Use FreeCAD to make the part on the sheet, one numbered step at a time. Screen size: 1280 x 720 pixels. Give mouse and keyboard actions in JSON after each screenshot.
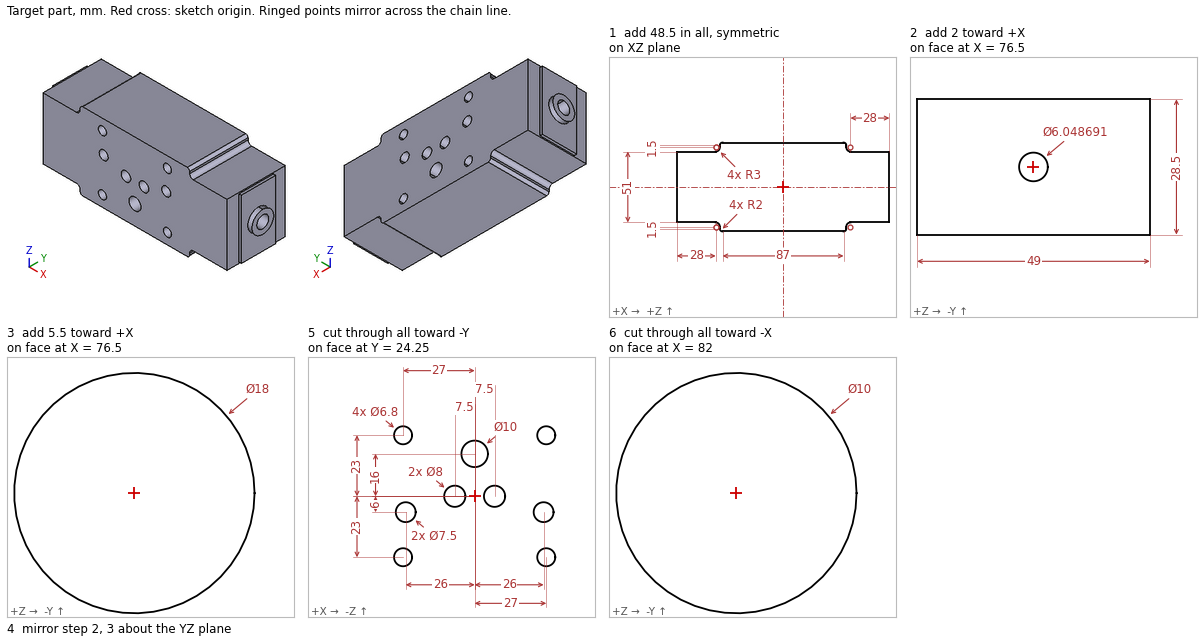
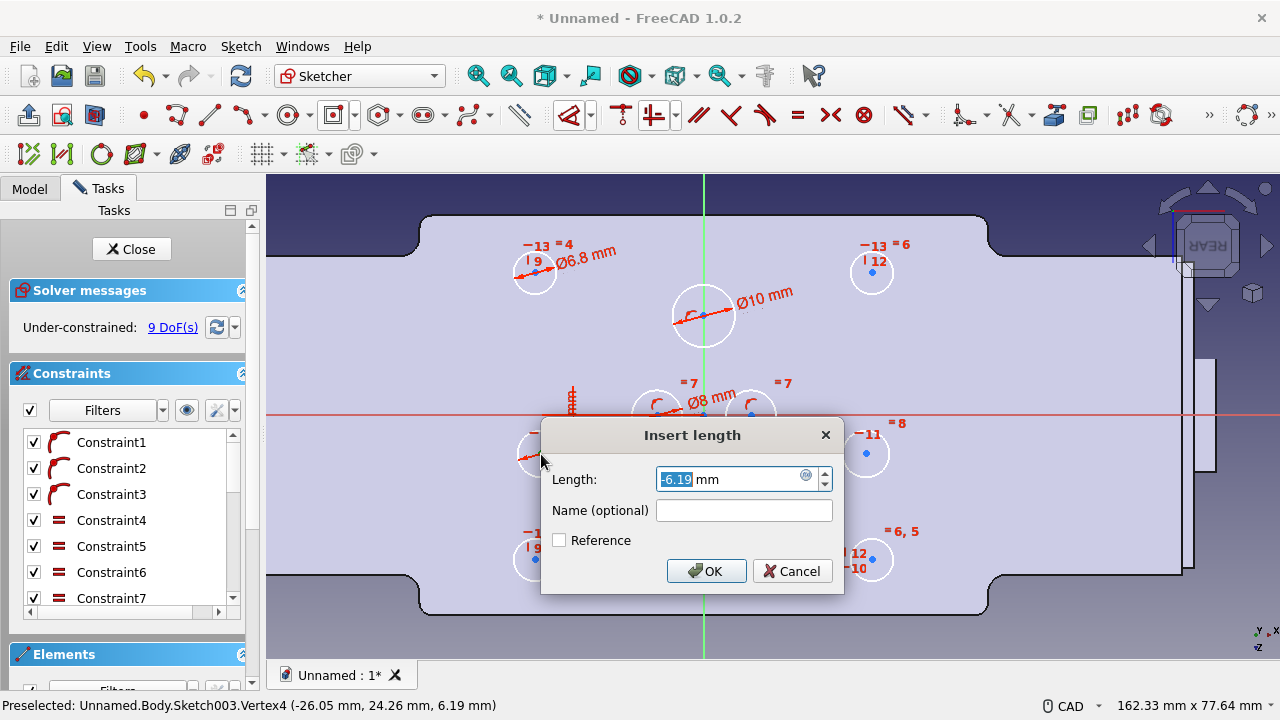
{"action": "type", "text": "-6"}
{"action": "key", "text": "Return"}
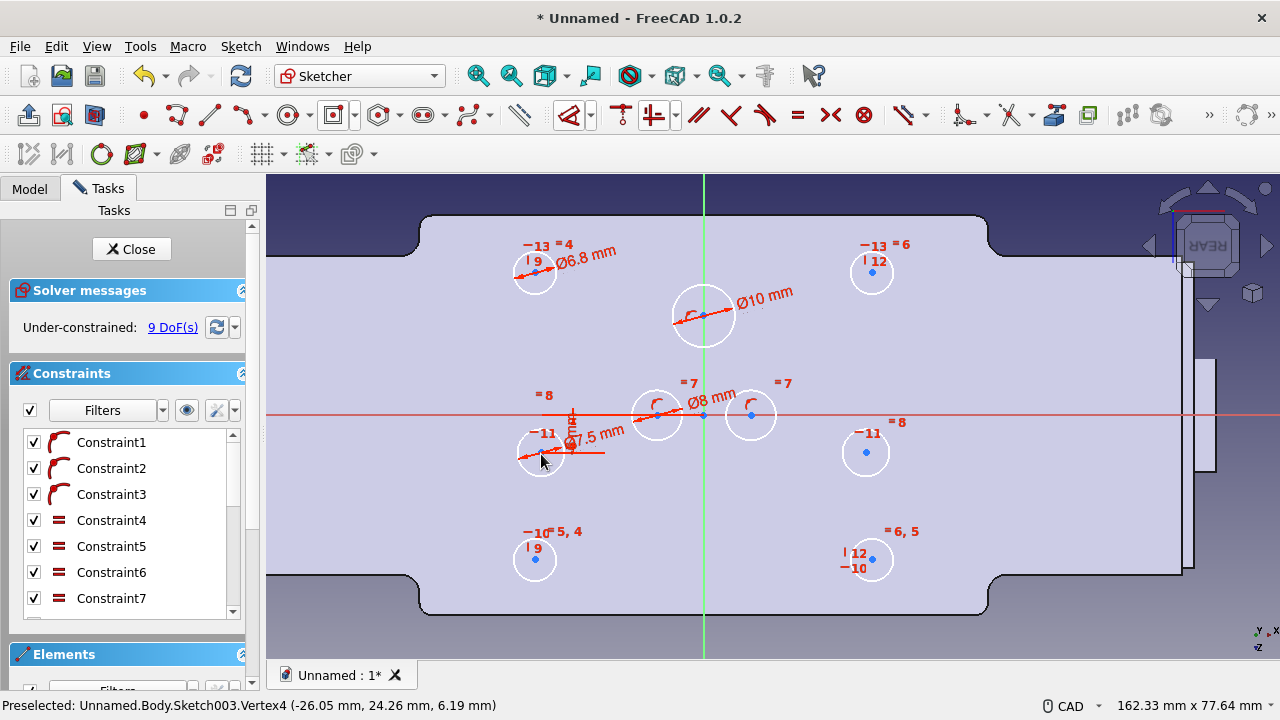
{"action": "left_click", "coordinate": [535, 273]}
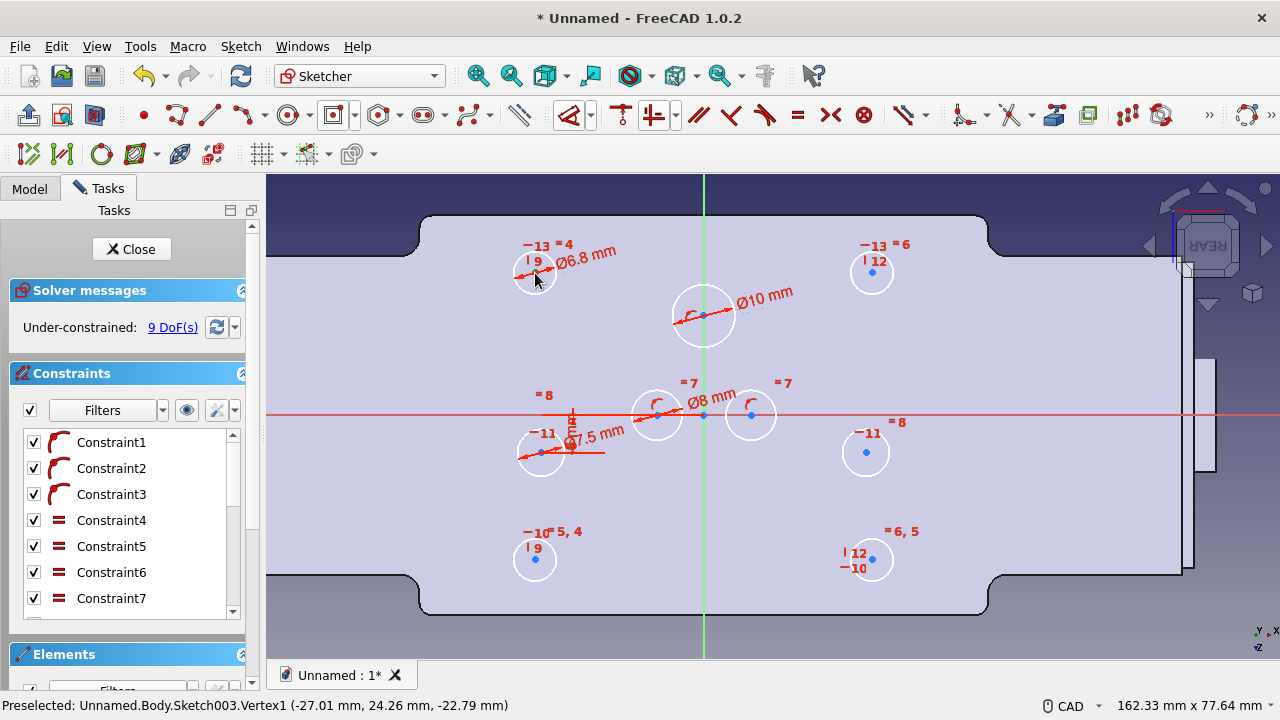
{"action": "key", "text": "l"}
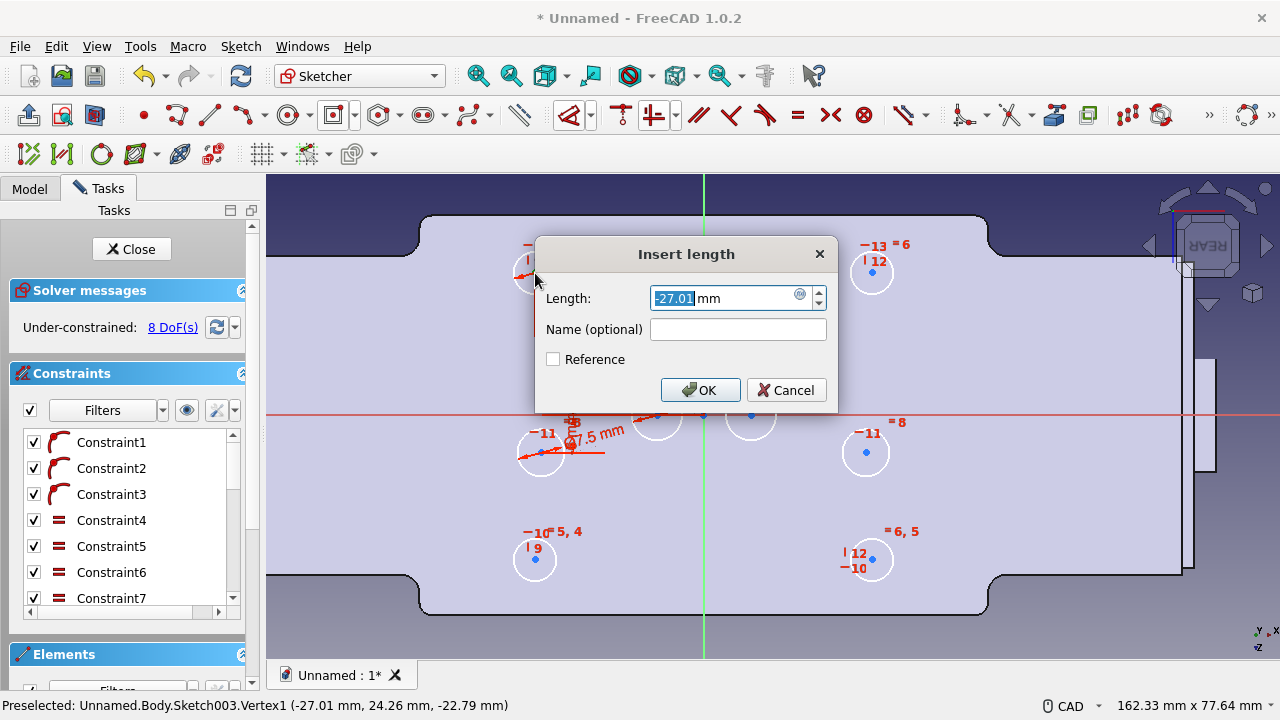
{"action": "type", "text": "-27"}
{"action": "key", "text": "Return"}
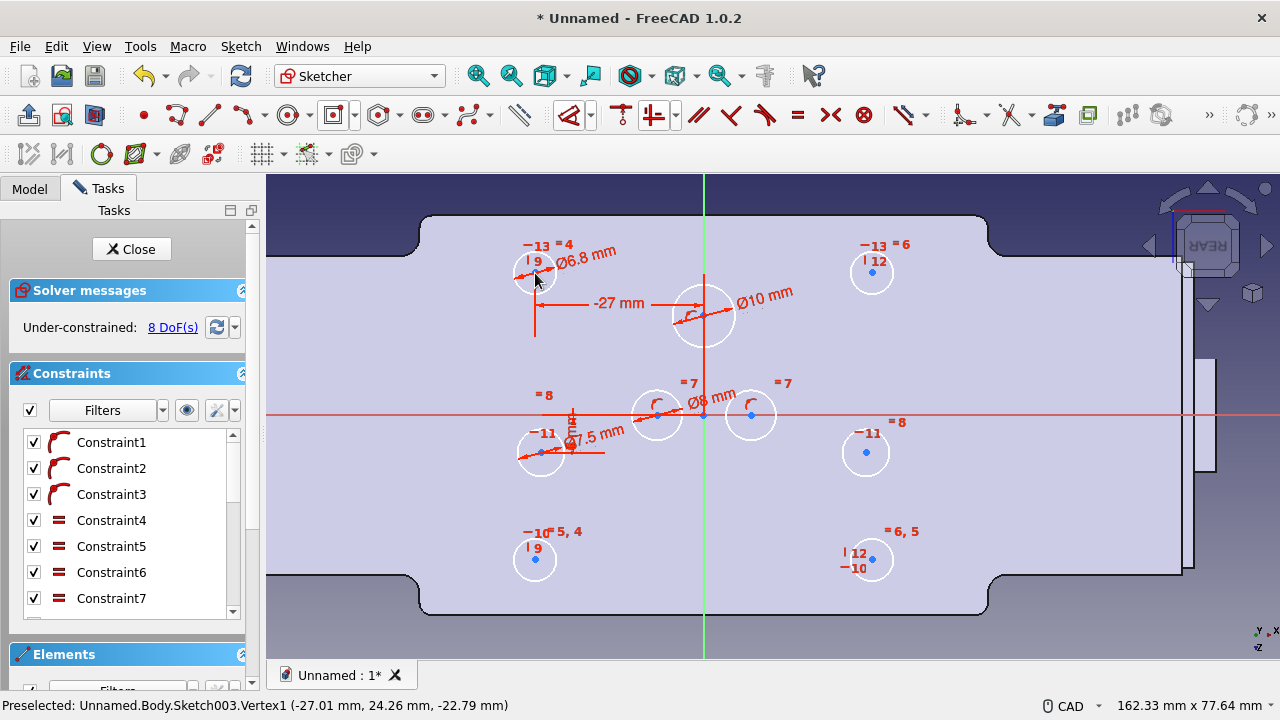
{"action": "left_click", "coordinate": [535, 273]}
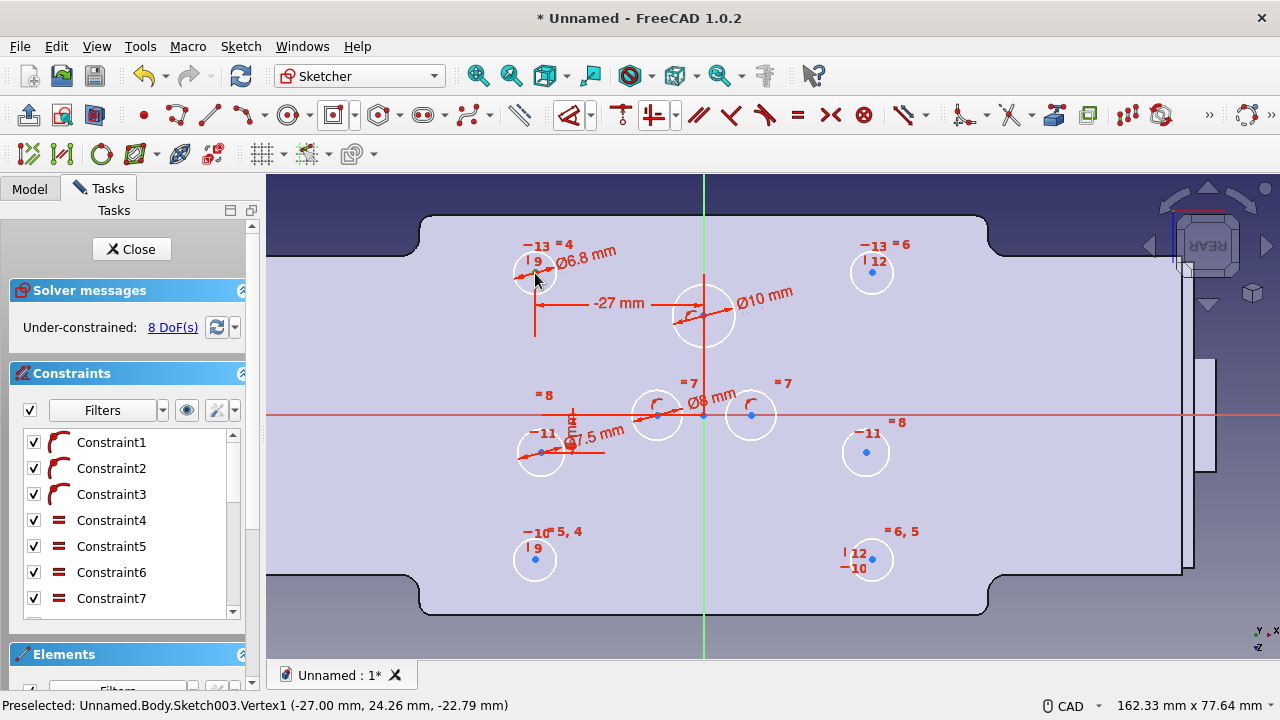
{"action": "left_click", "coordinate": [590, 116]}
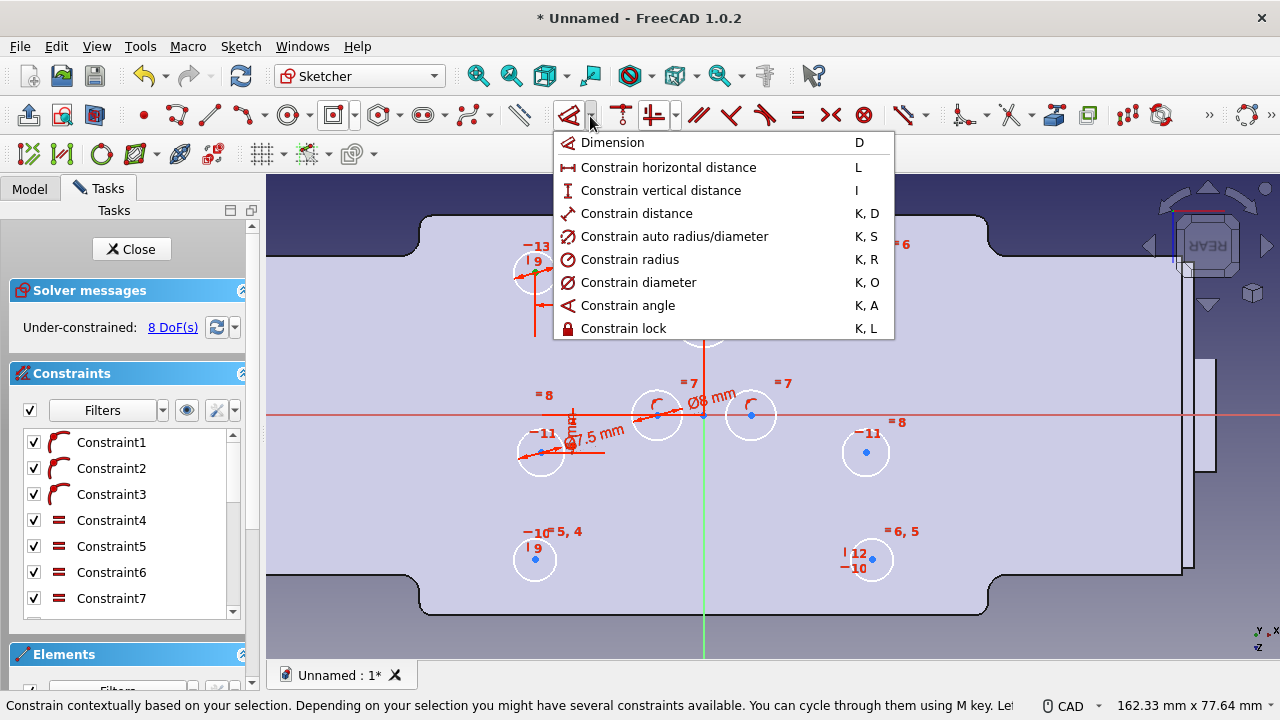
{"action": "left_click", "coordinate": [724, 190]}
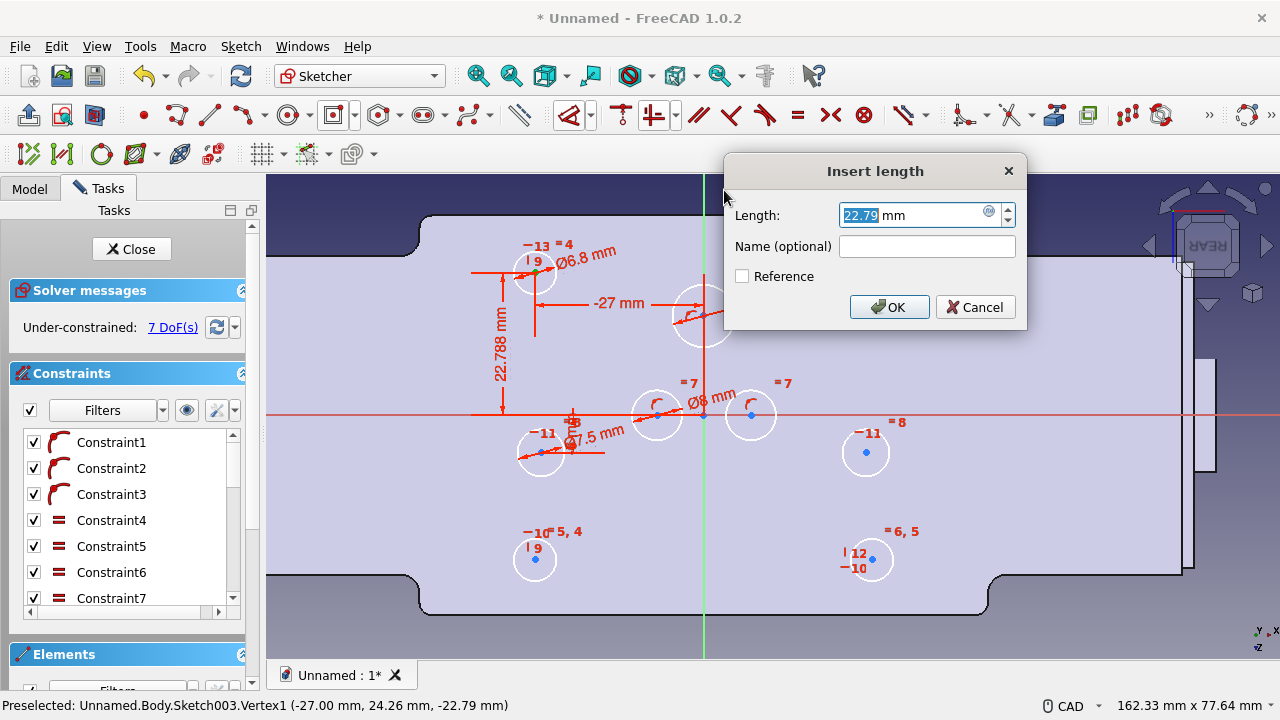
{"action": "type", "text": "23"}
{"action": "key", "text": "Return"}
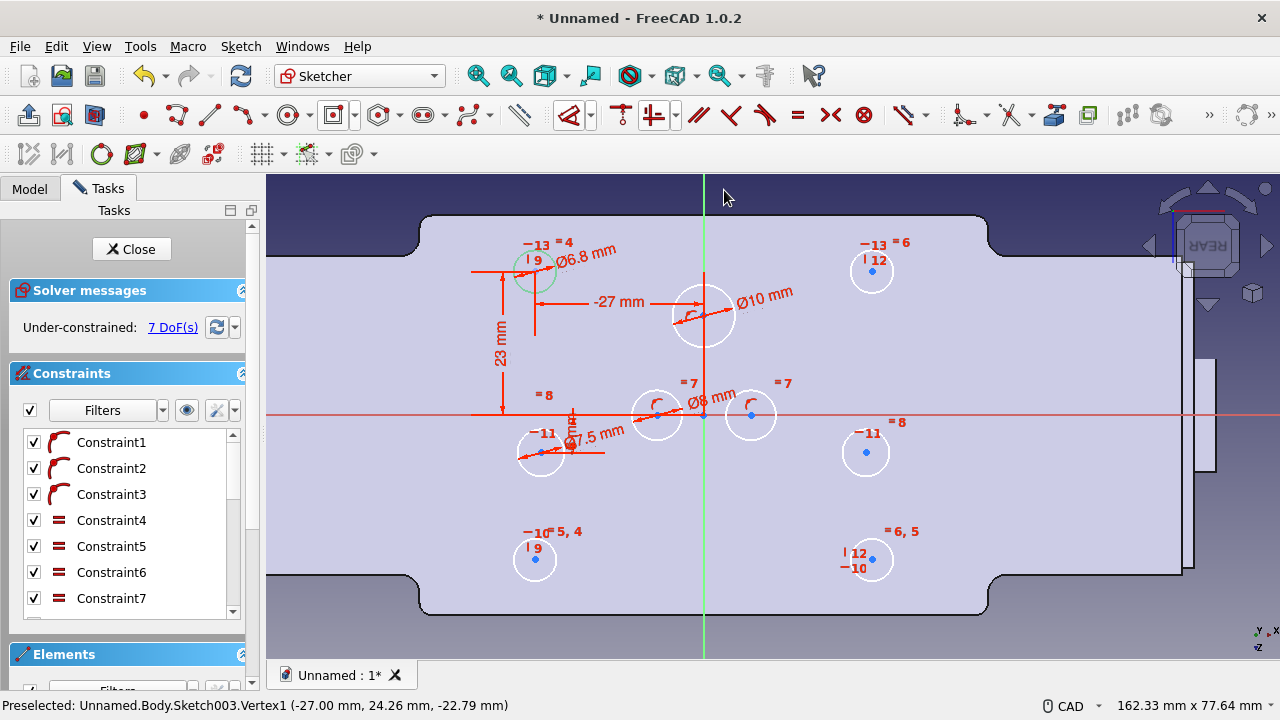
{"action": "left_click", "coordinate": [704, 316]}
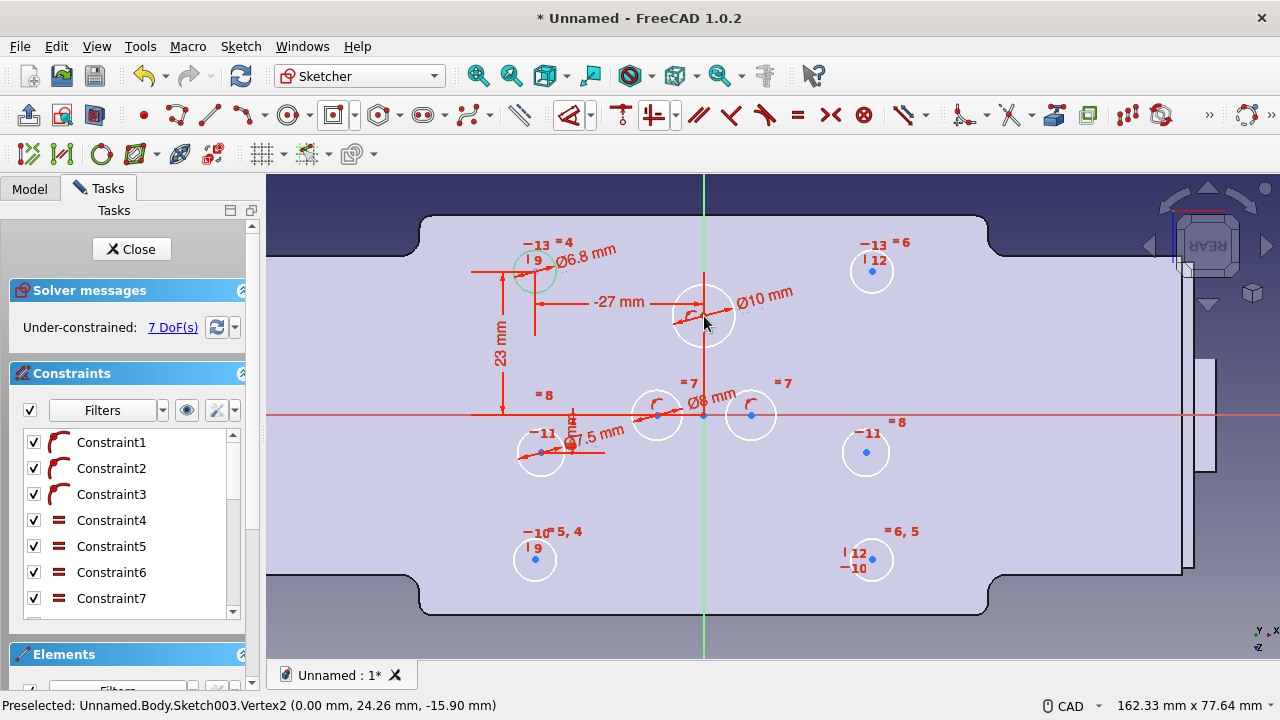
{"action": "left_click", "coordinate": [590, 116]}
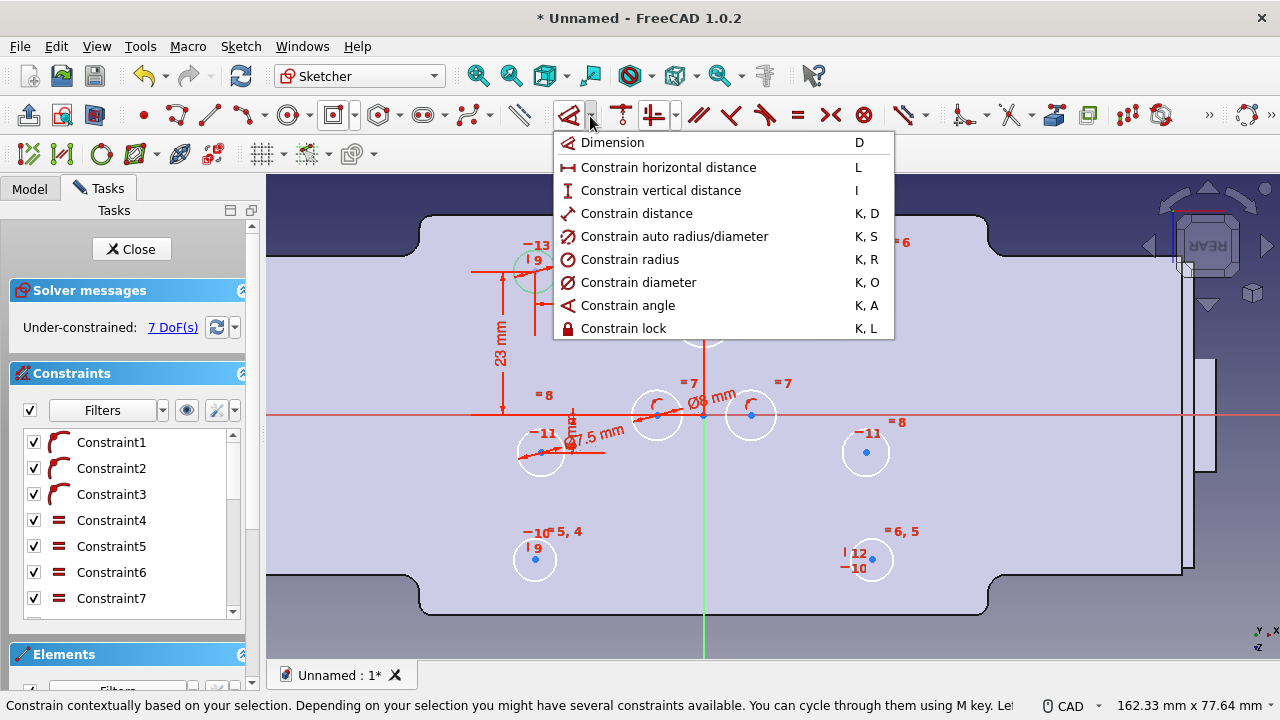
{"action": "left_click", "coordinate": [724, 190]}